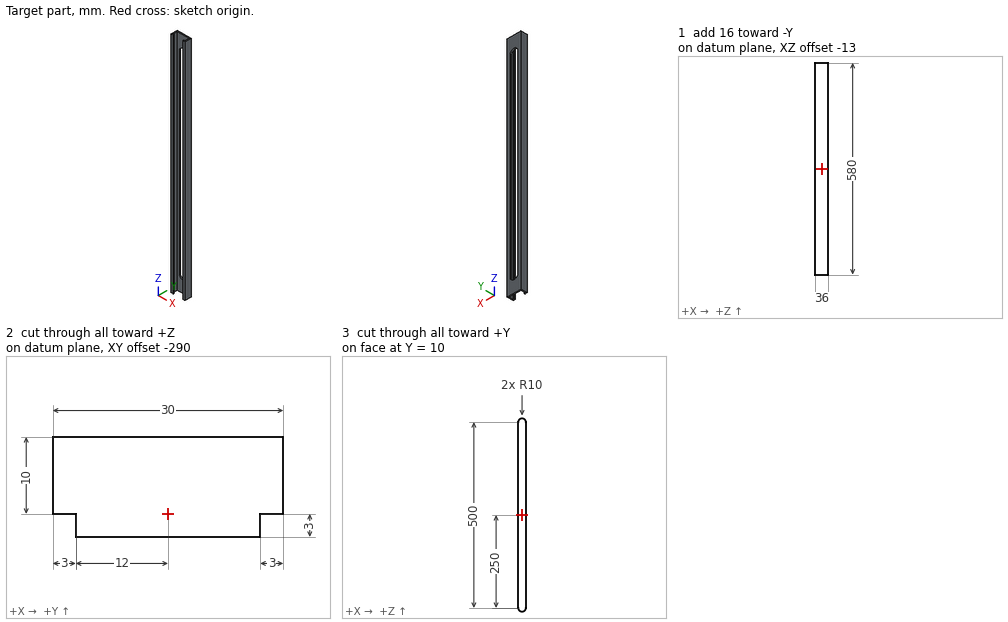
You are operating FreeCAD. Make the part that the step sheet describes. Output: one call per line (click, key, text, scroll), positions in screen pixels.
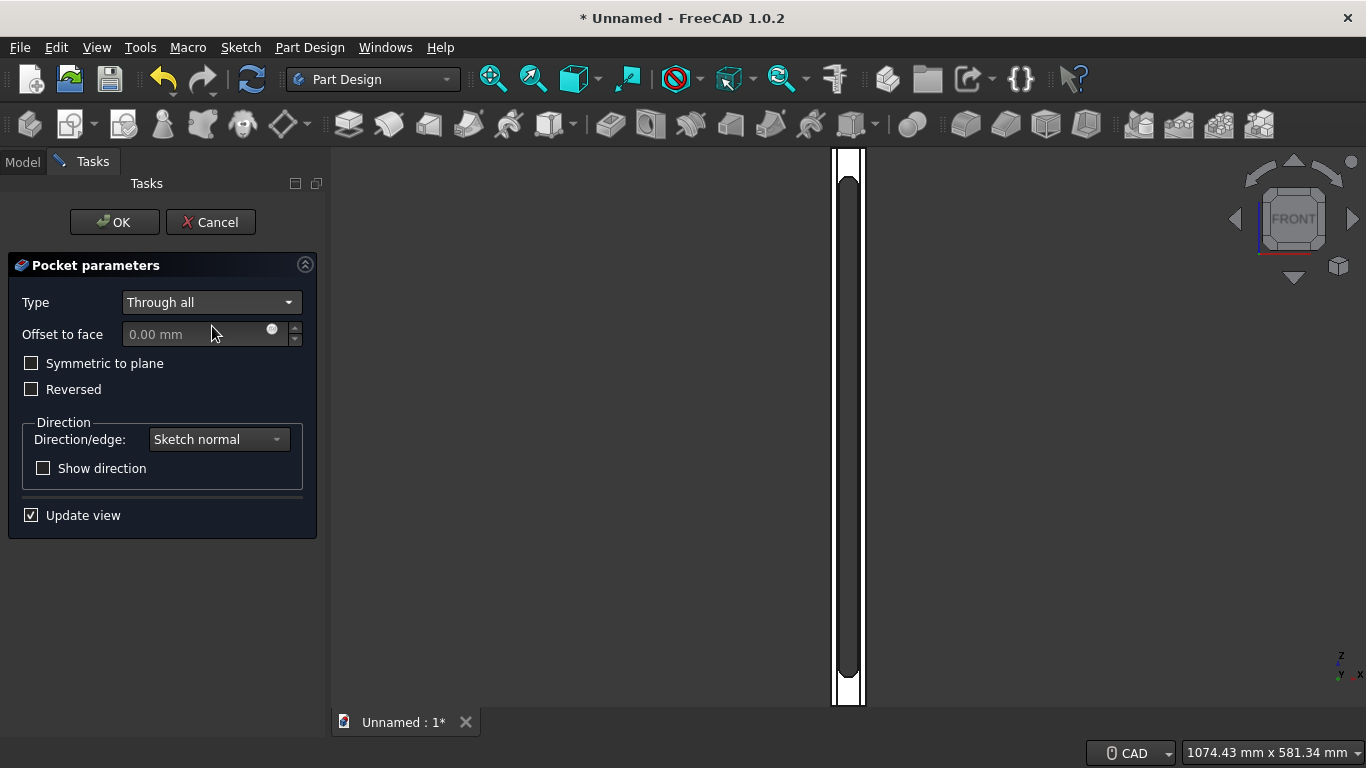
click(115, 222)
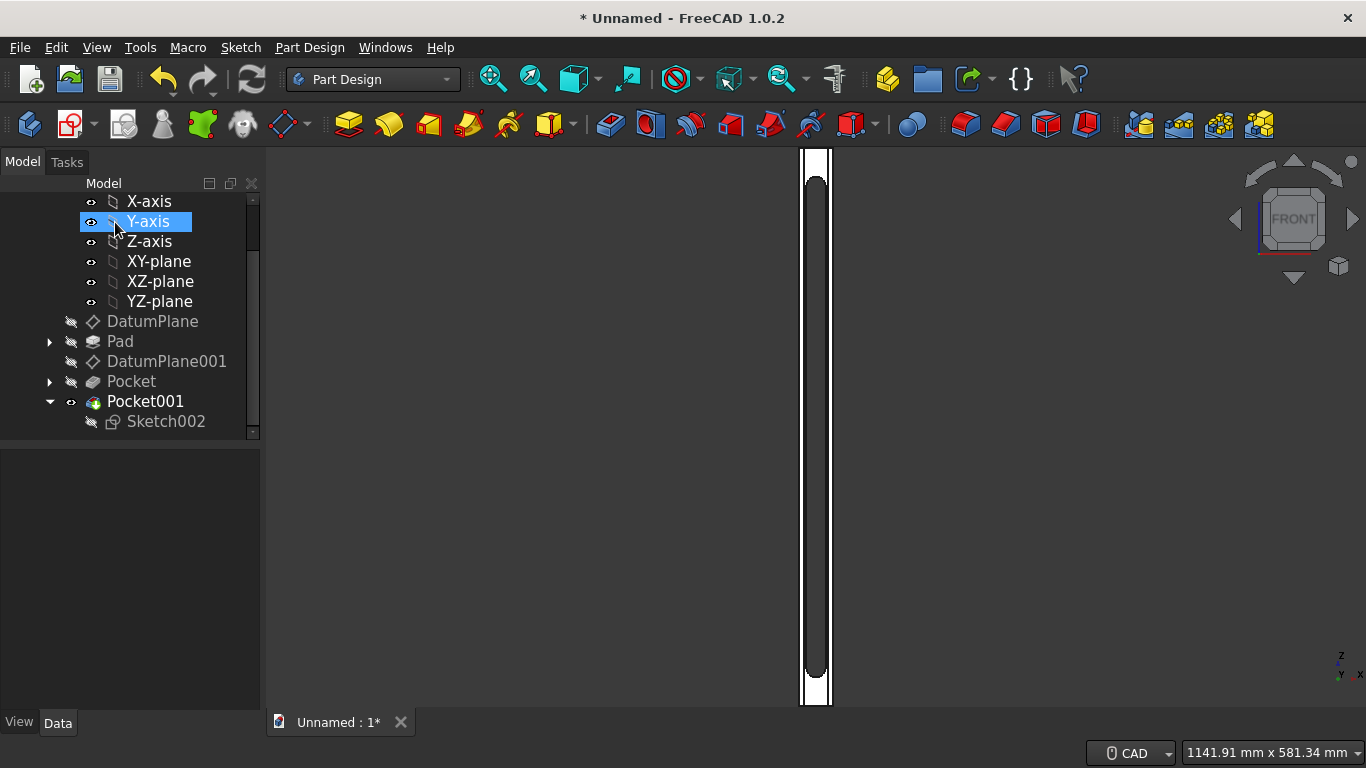
key(0)